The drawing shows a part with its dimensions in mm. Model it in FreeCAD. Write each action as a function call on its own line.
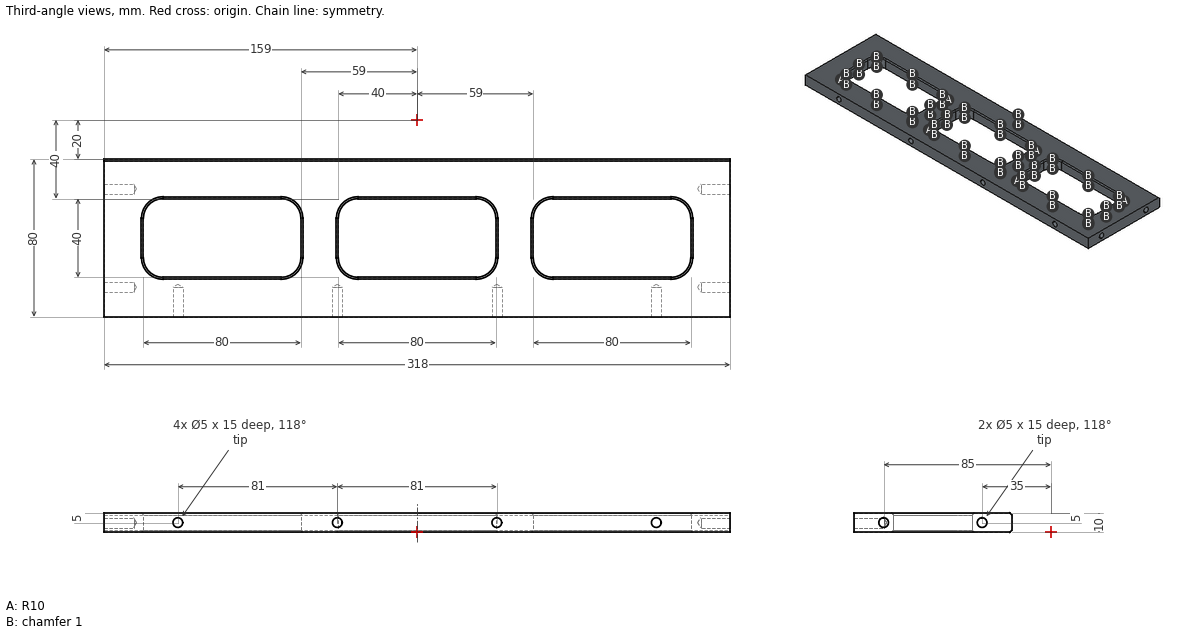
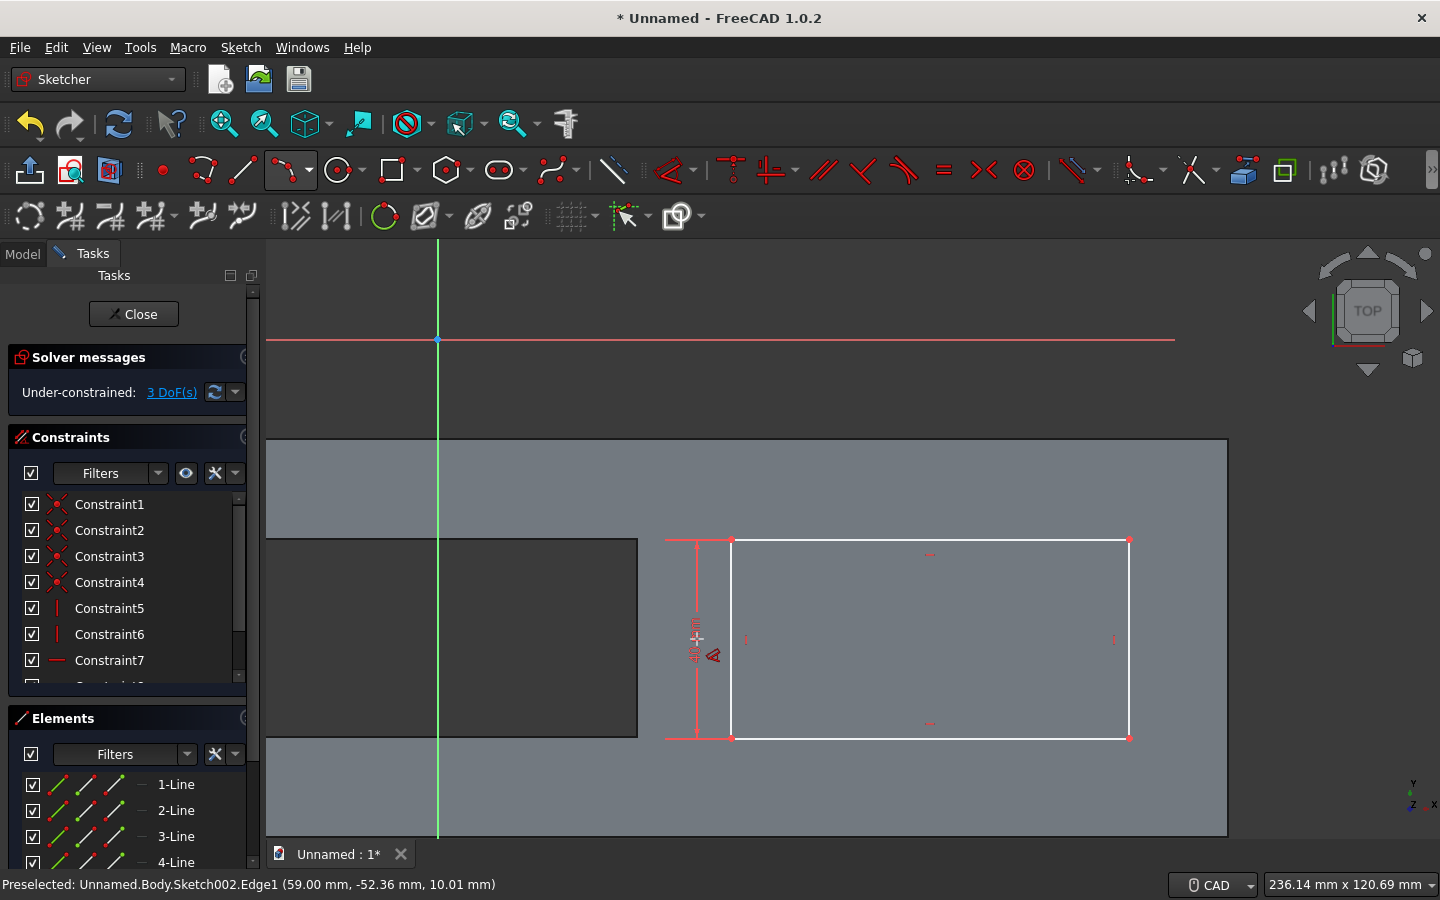
click(850, 739)
click(930, 773)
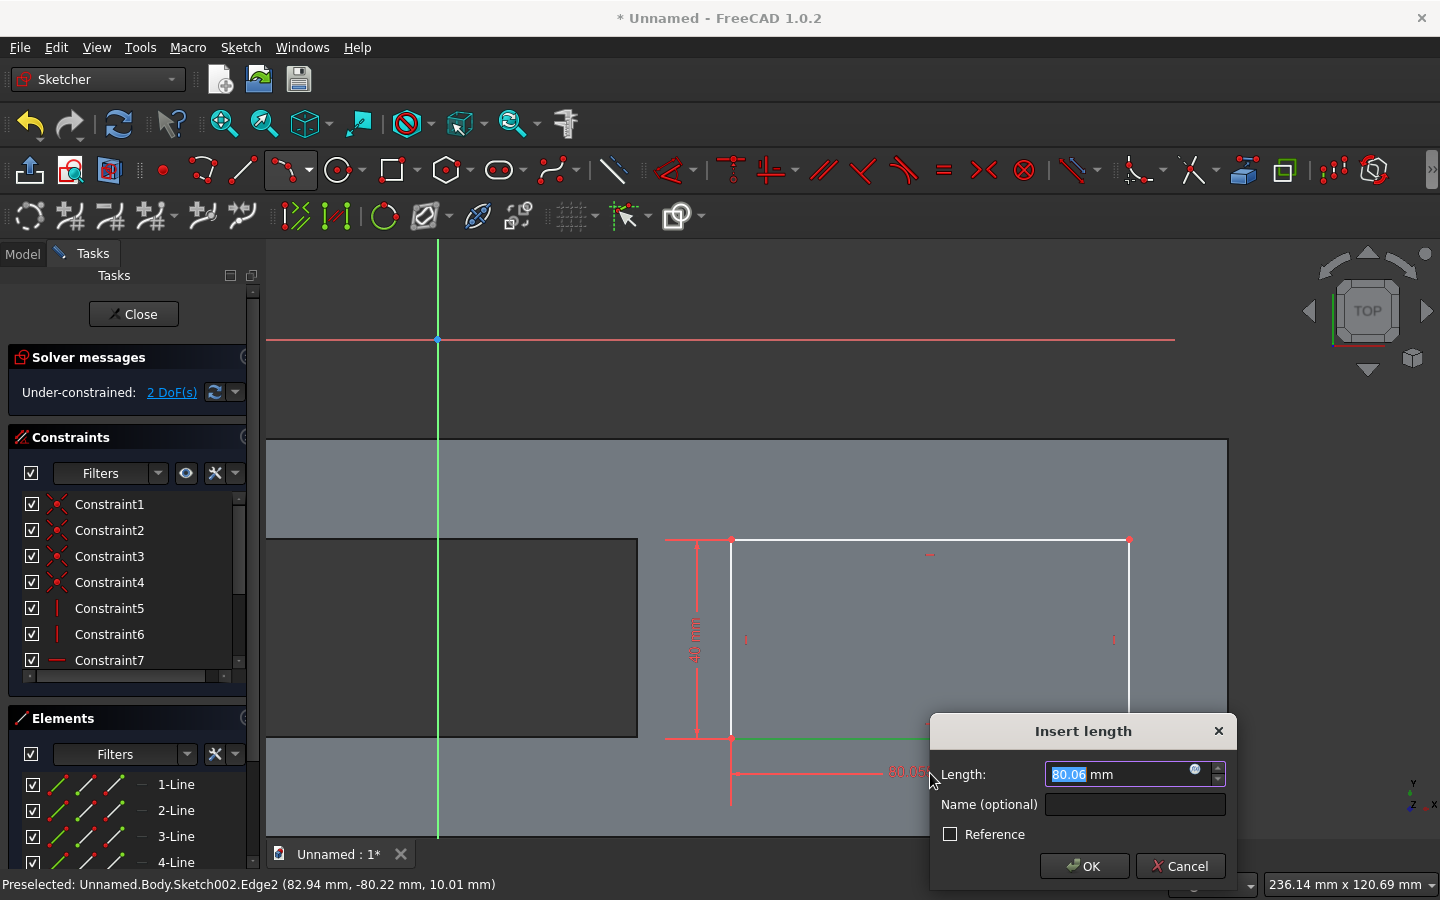
text(80)
key(Return)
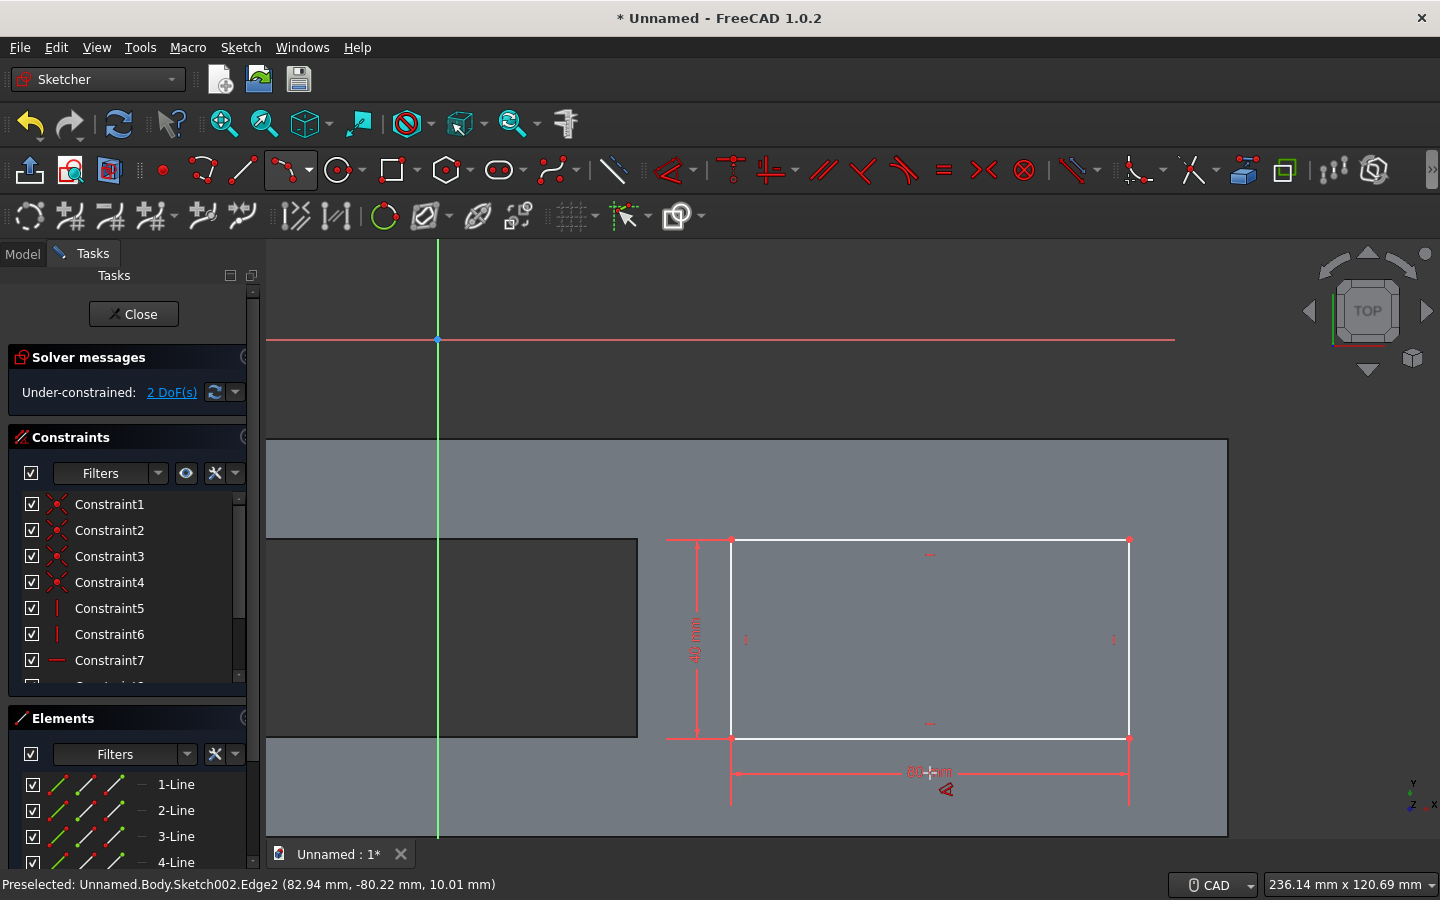
click(731, 540)
click(584, 306)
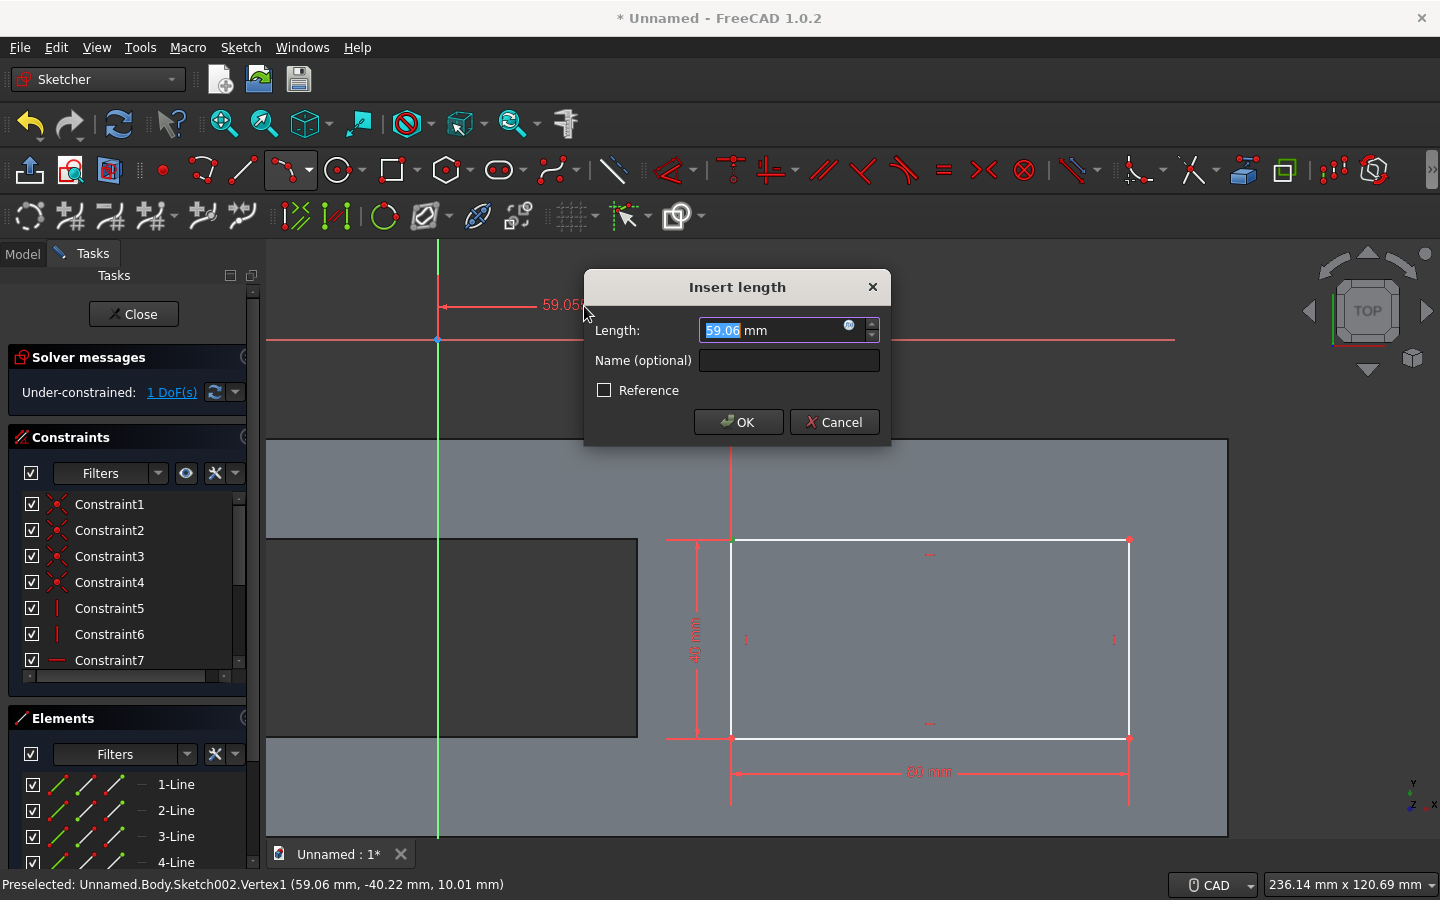
text(59)
key(Return)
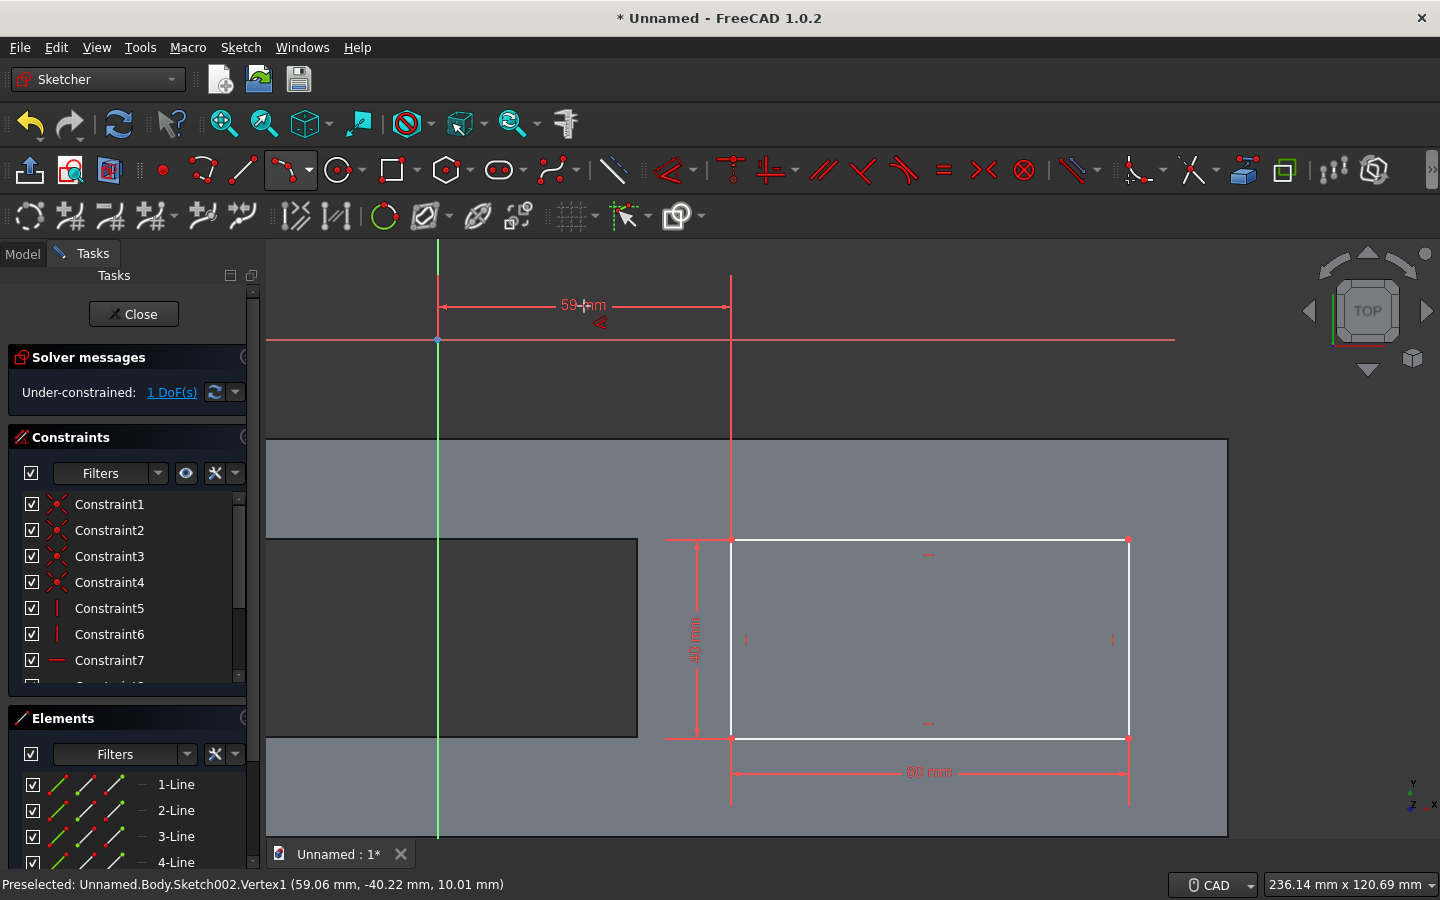
click(731, 540)
click(404, 440)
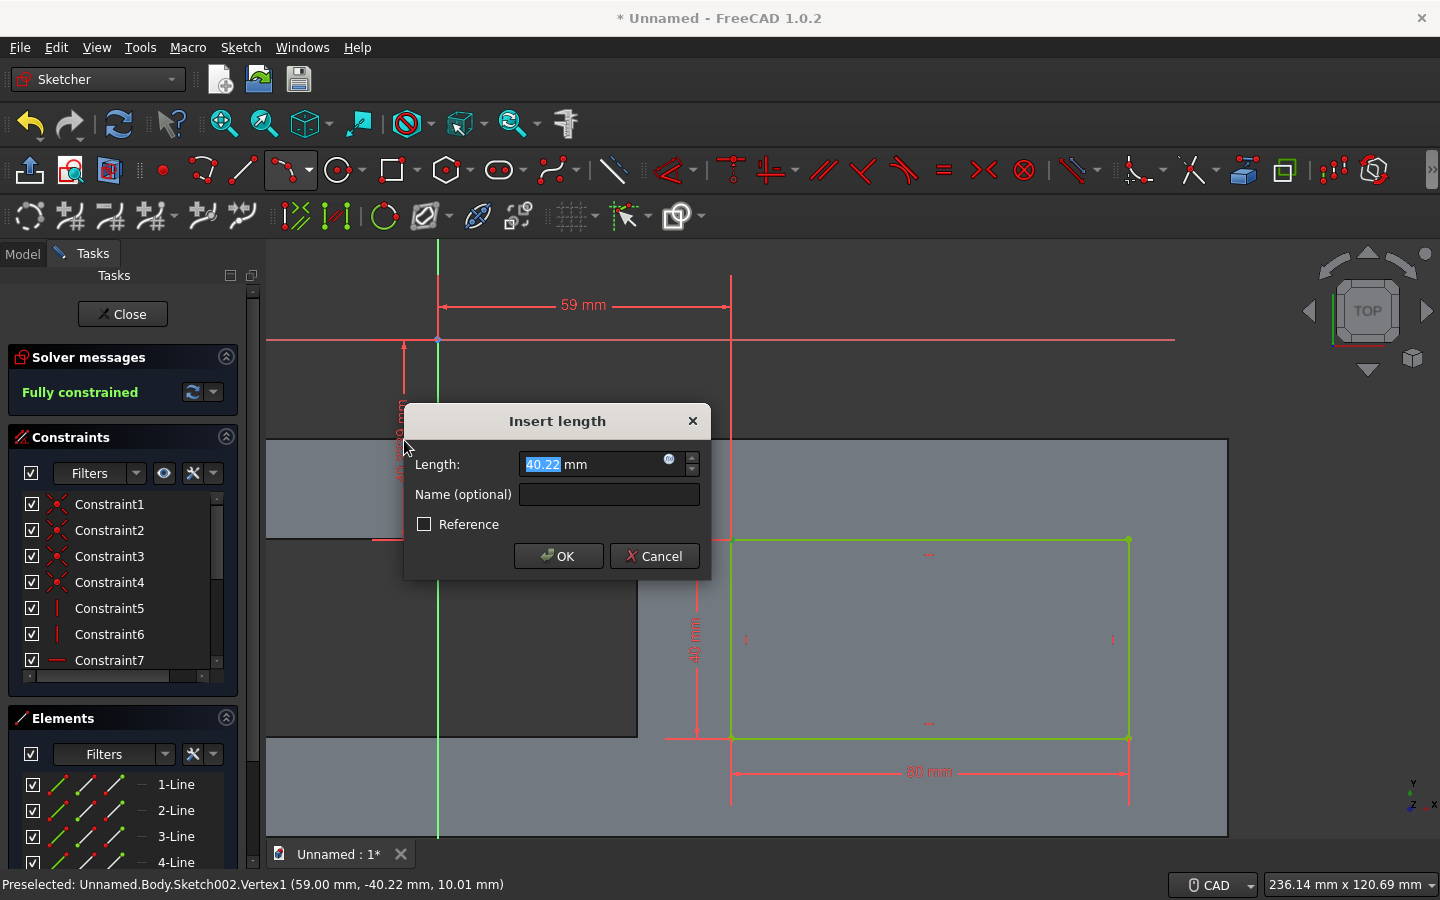
text(40)
key(Return)
key(Escape)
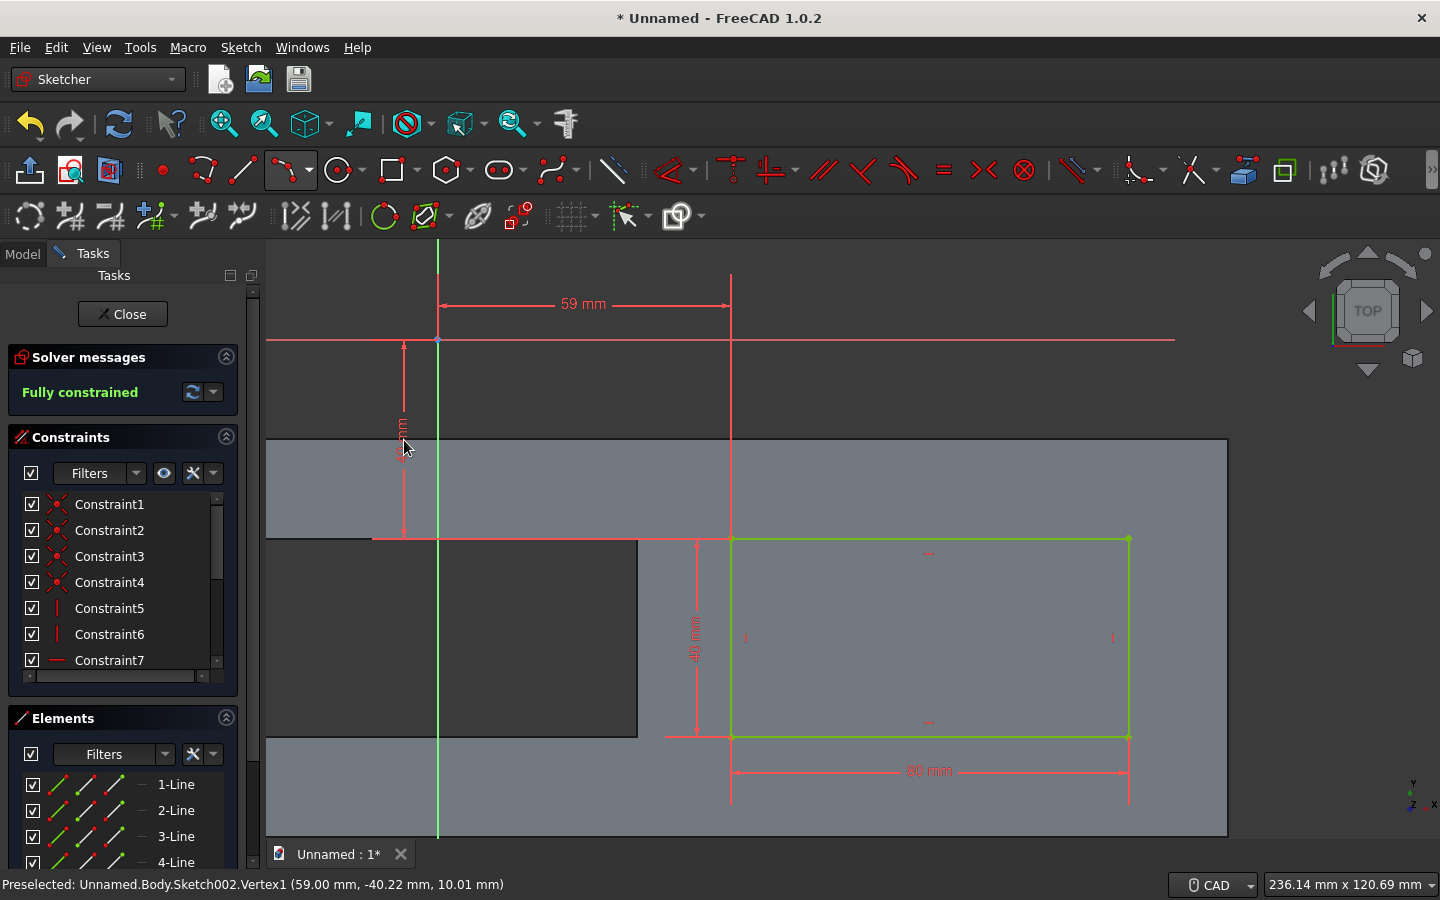
click(123, 314)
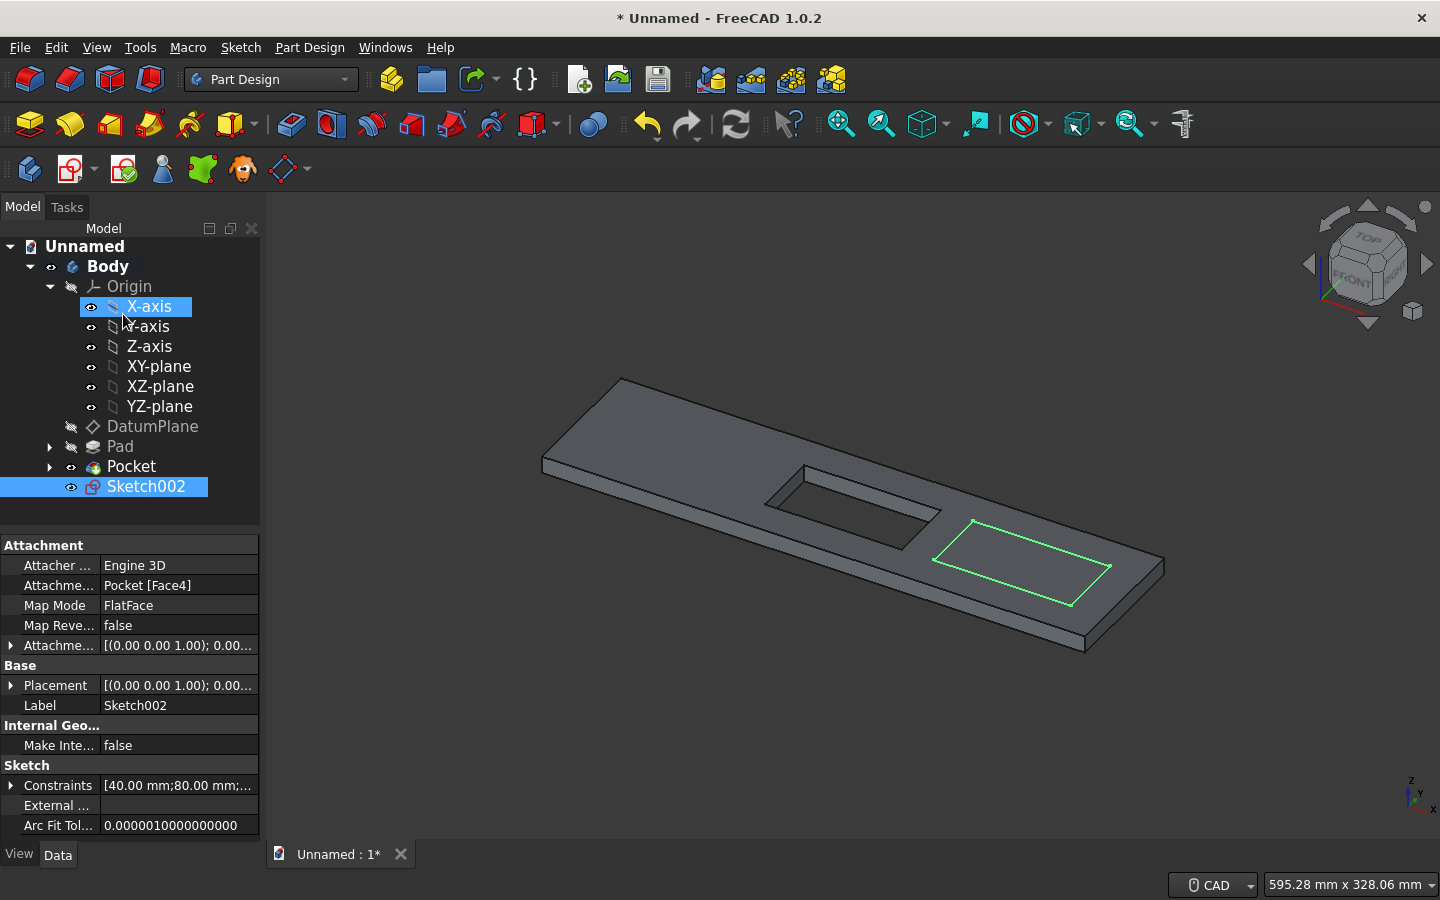
click(292, 124)